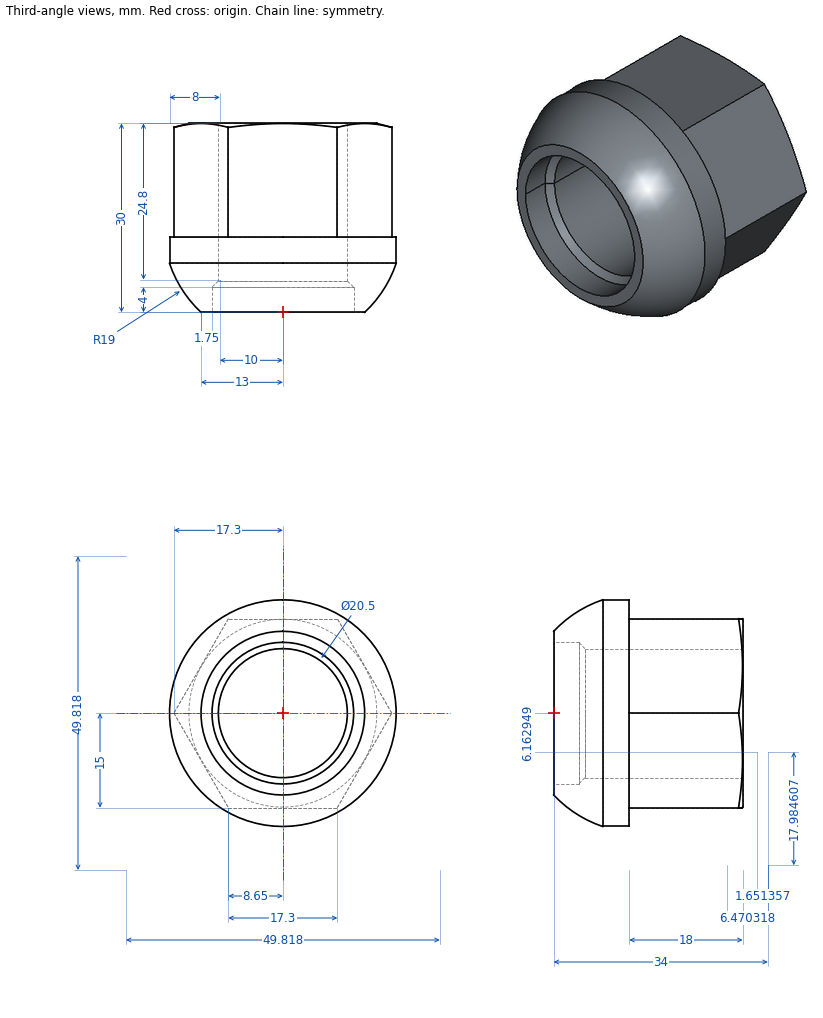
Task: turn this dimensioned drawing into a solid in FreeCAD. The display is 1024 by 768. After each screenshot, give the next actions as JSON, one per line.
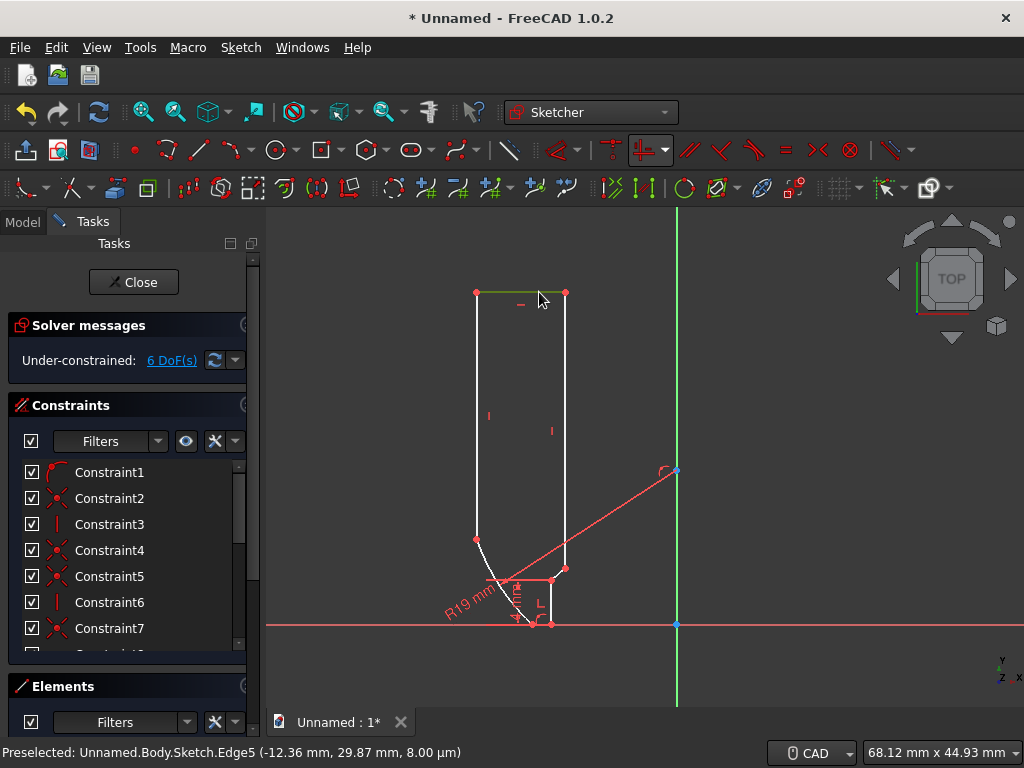
{"action": "key", "text": "l"}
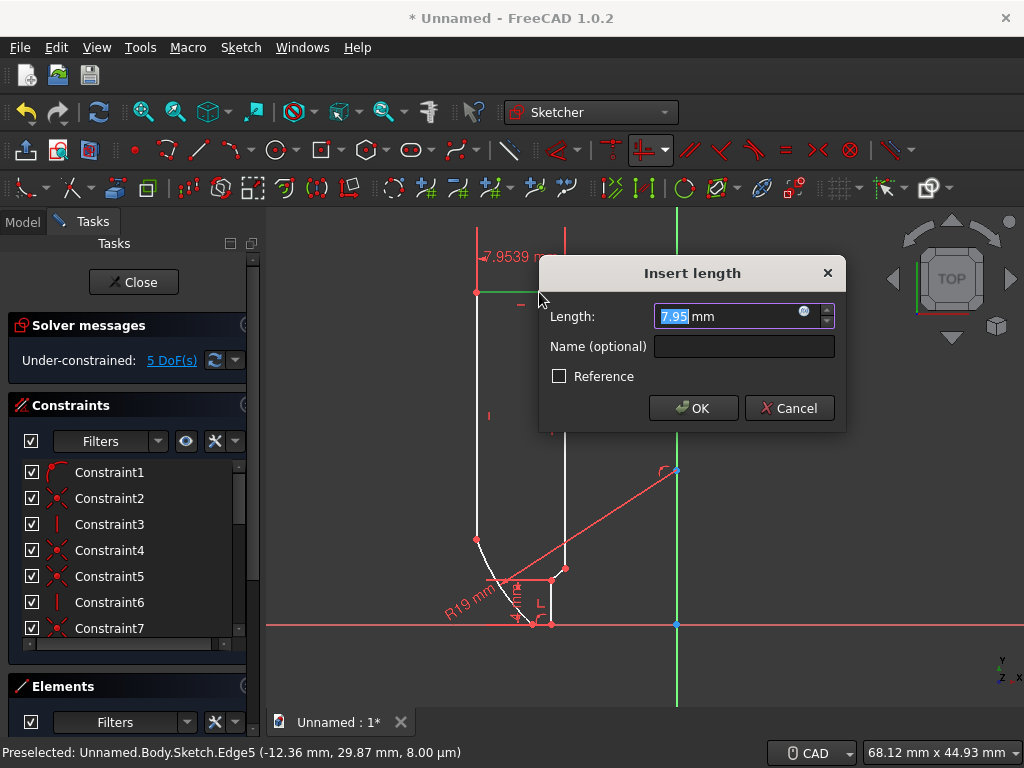
{"action": "type", "text": "8"}
{"action": "key", "text": "Return"}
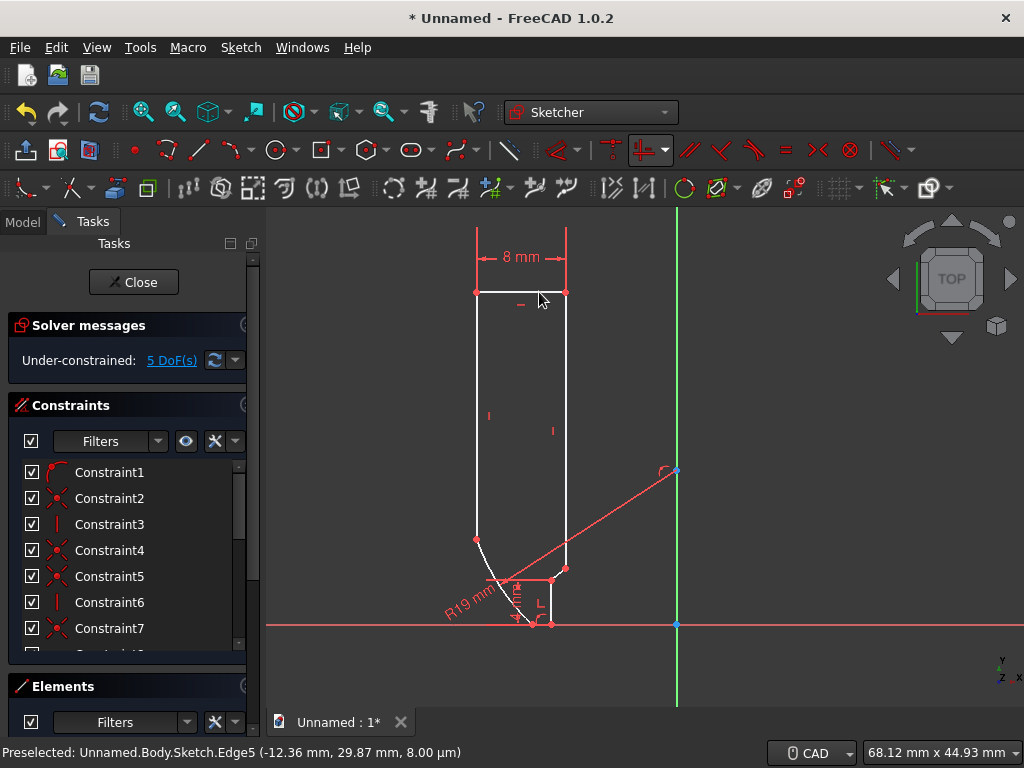
{"action": "left_click", "coordinate": [532, 625]}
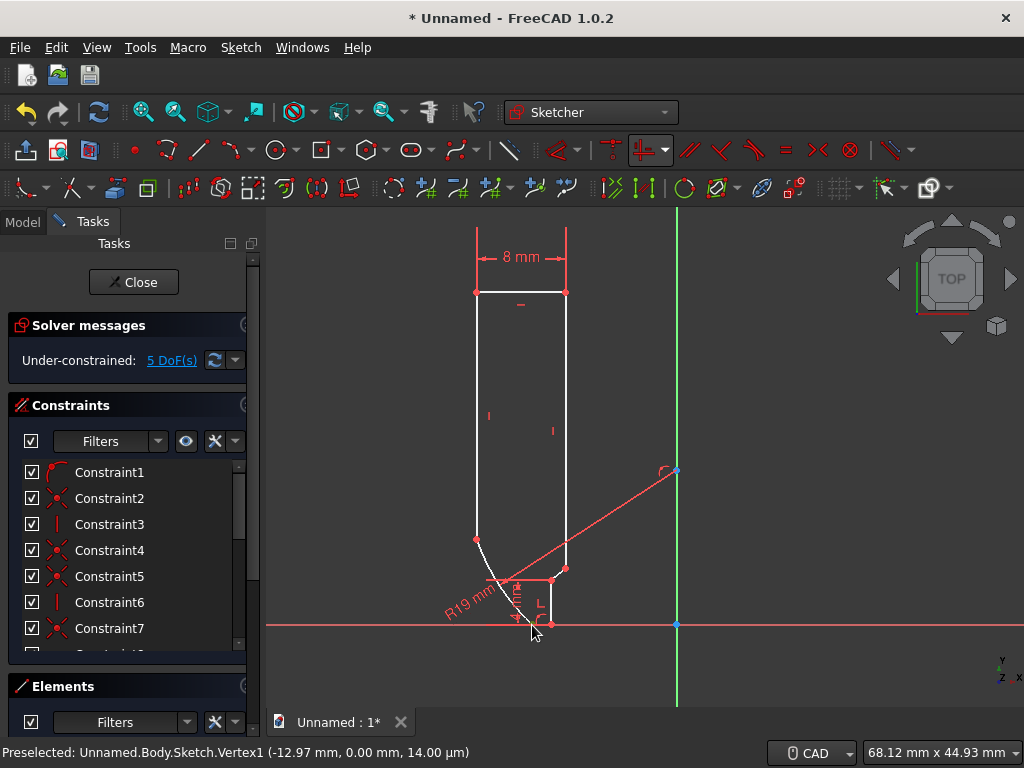
{"action": "key", "text": "l"}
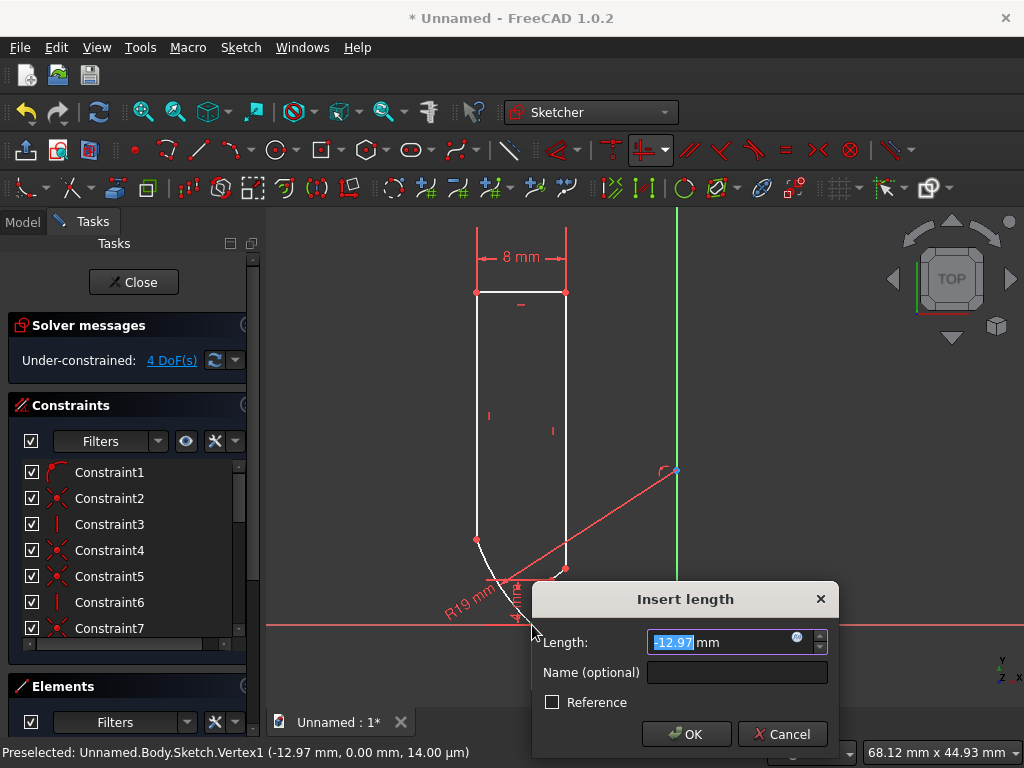
{"action": "type", "text": "-13"}
{"action": "key", "text": "Return"}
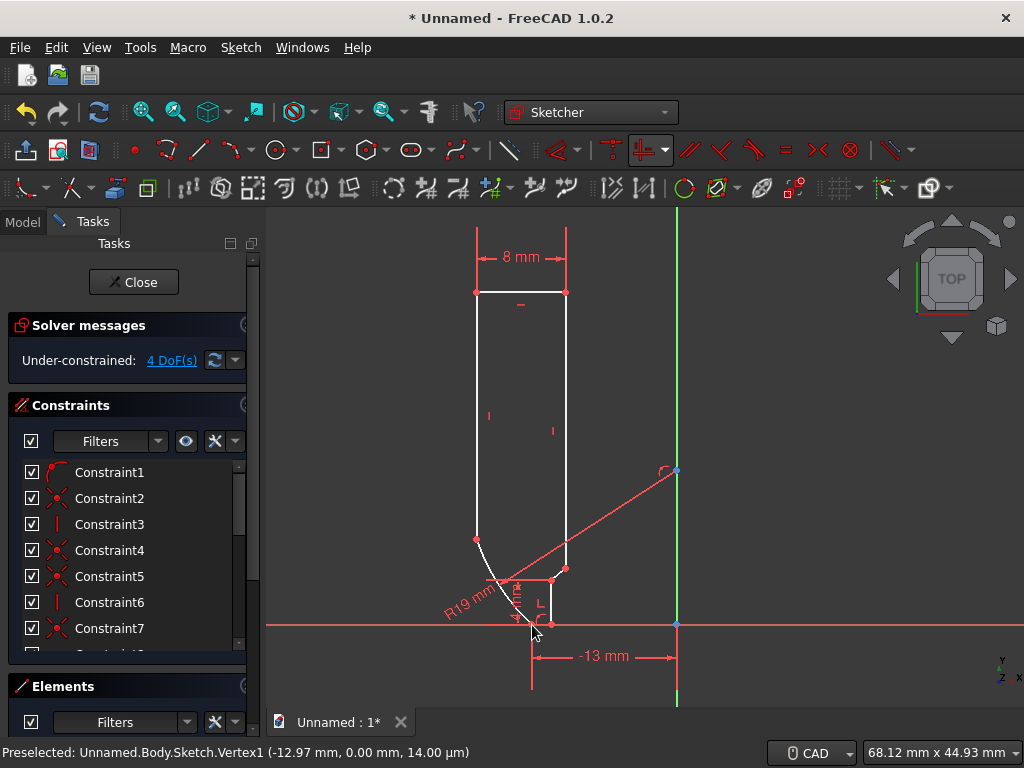
{"action": "left_click", "coordinate": [566, 568]}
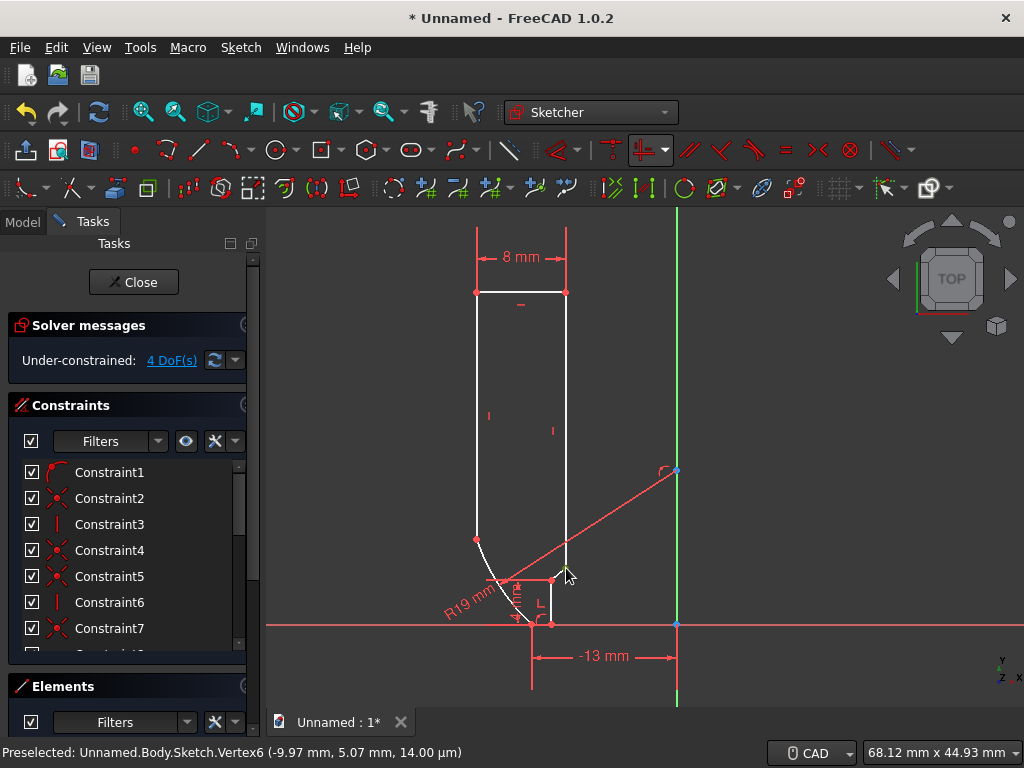
{"action": "key", "text": "l"}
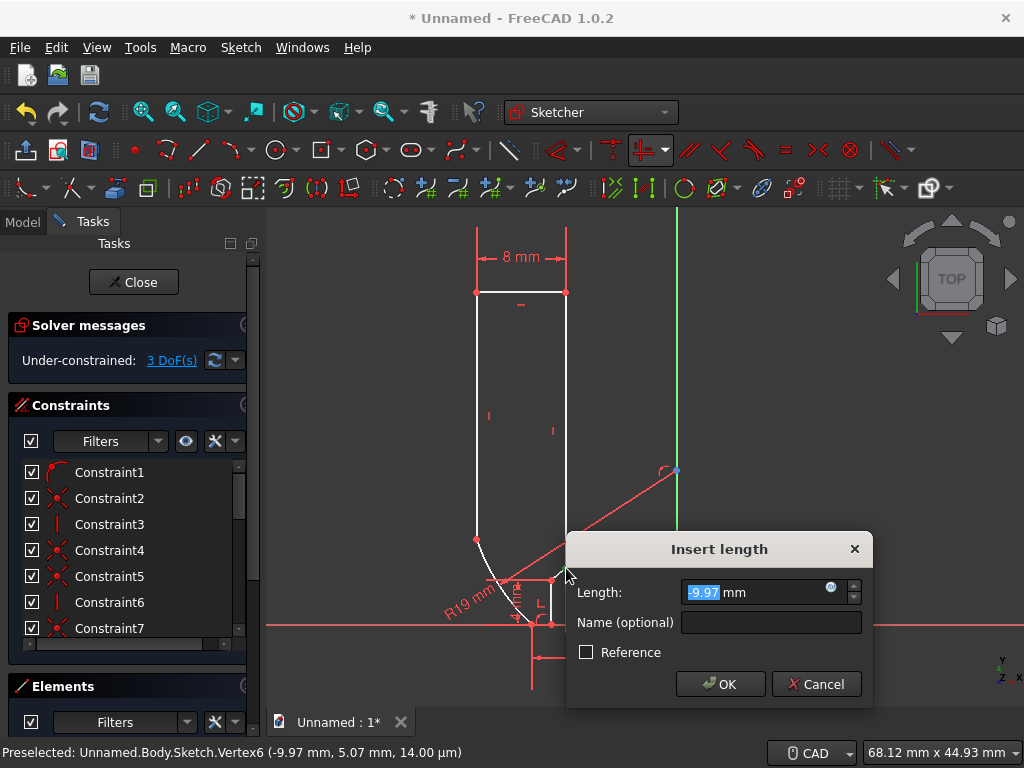
{"action": "type", "text": "-10"}
{"action": "key", "text": "Return"}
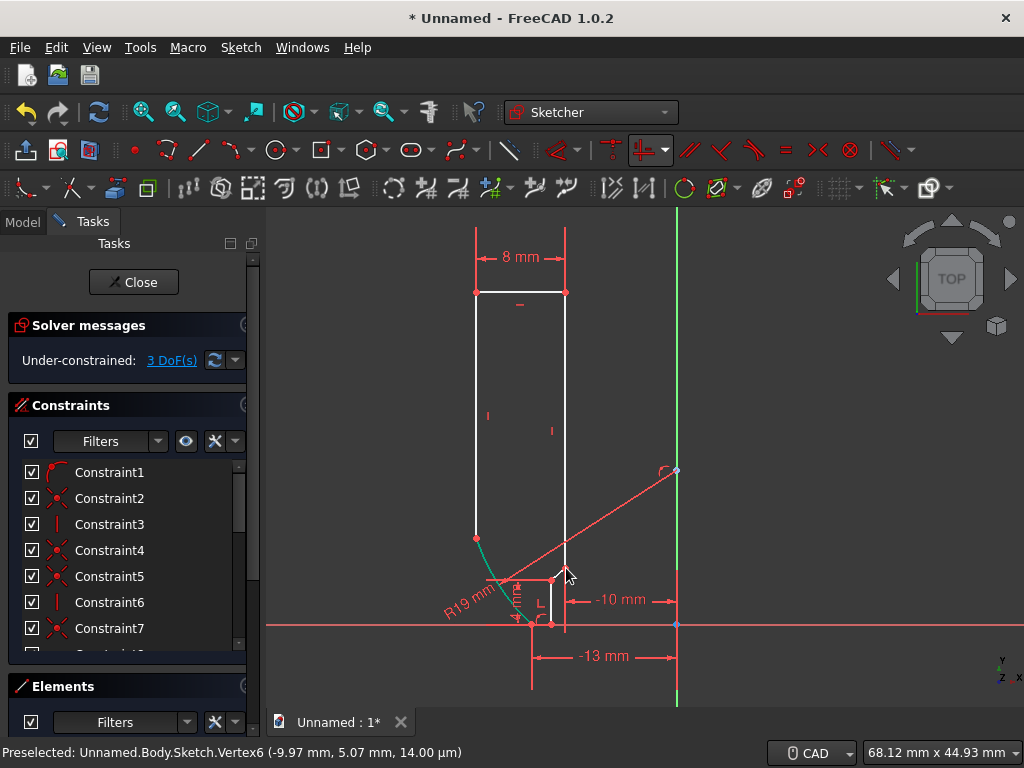
{"action": "left_click", "coordinate": [565, 292]}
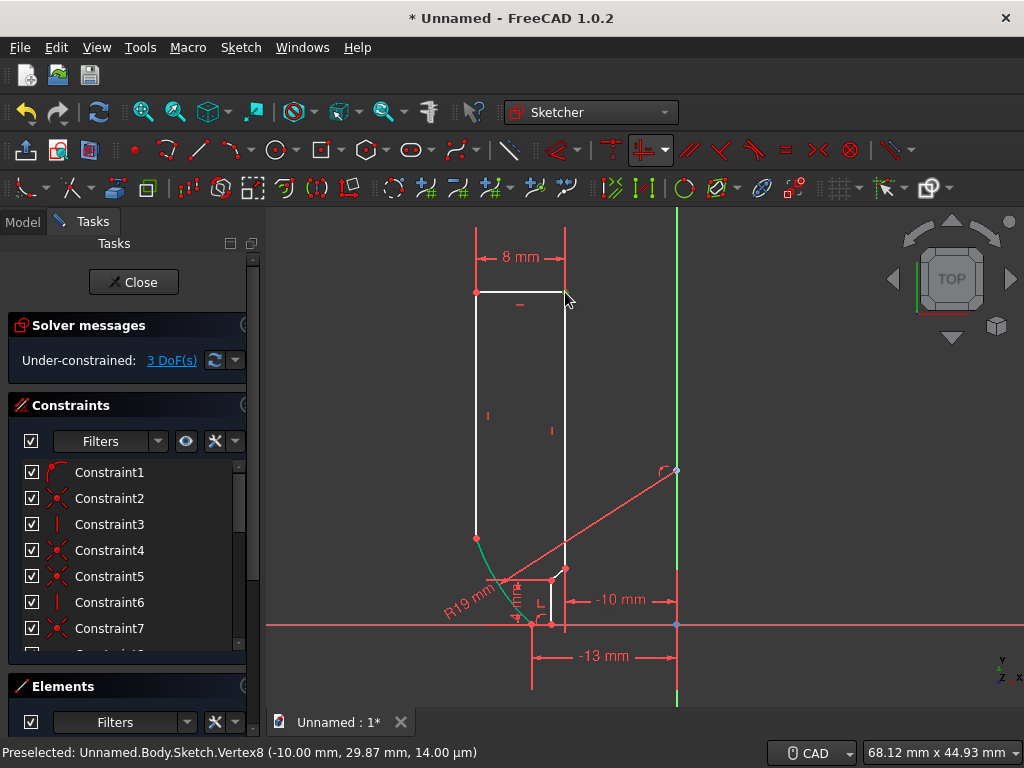
{"action": "key", "text": "i"}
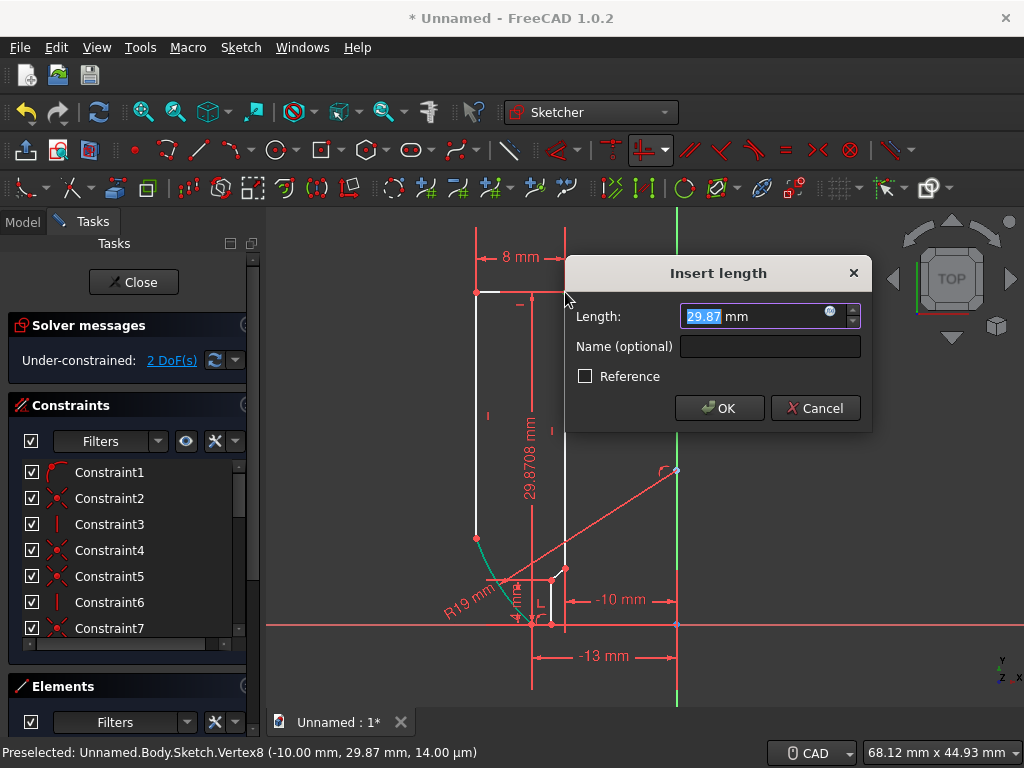
{"action": "type", "text": "30"}
{"action": "key", "text": "Return"}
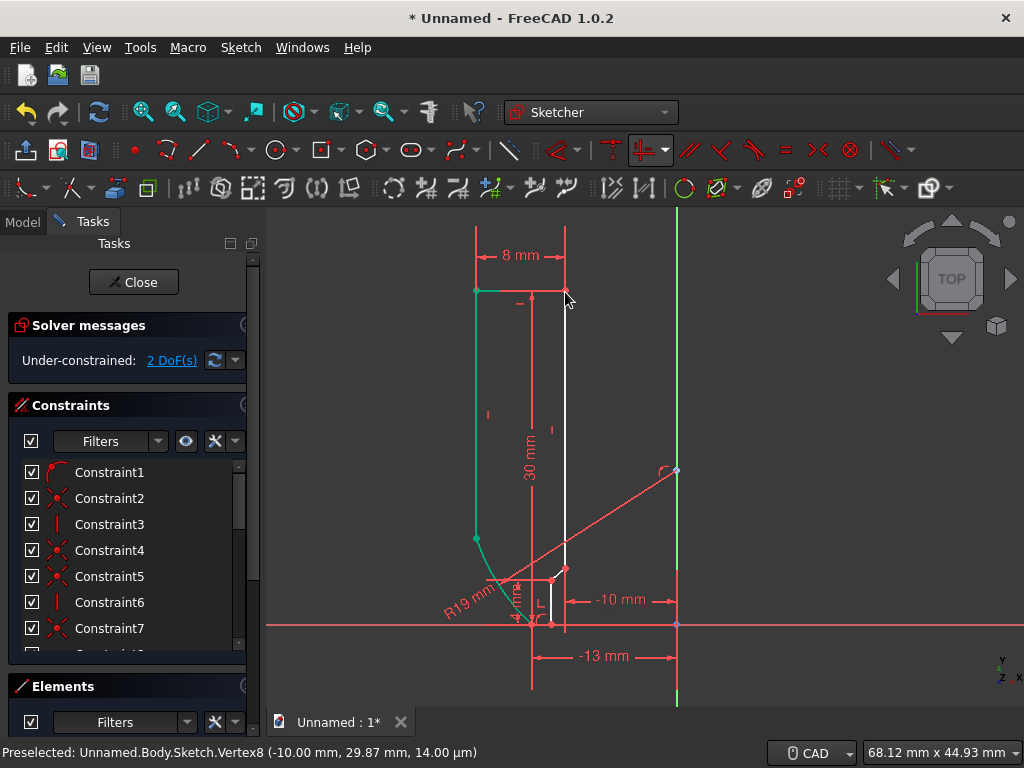
{"action": "scroll", "coordinate": [542, 625], "scroll_direction": "up", "scroll_amount": 4}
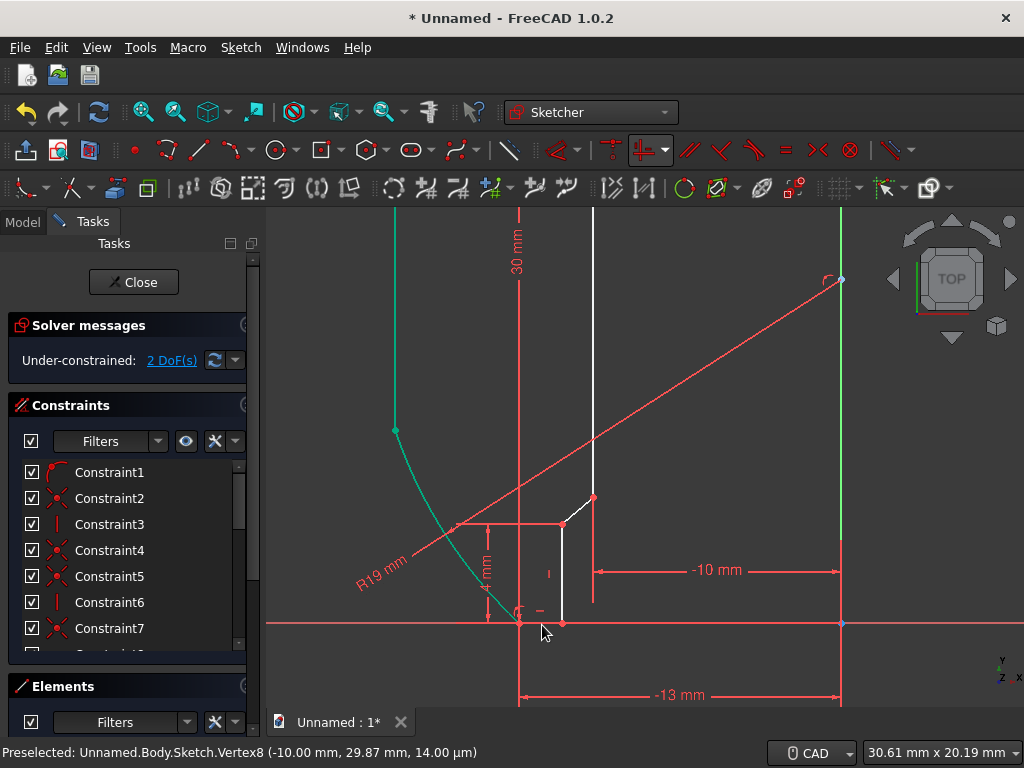
{"action": "left_click", "coordinate": [541, 623]}